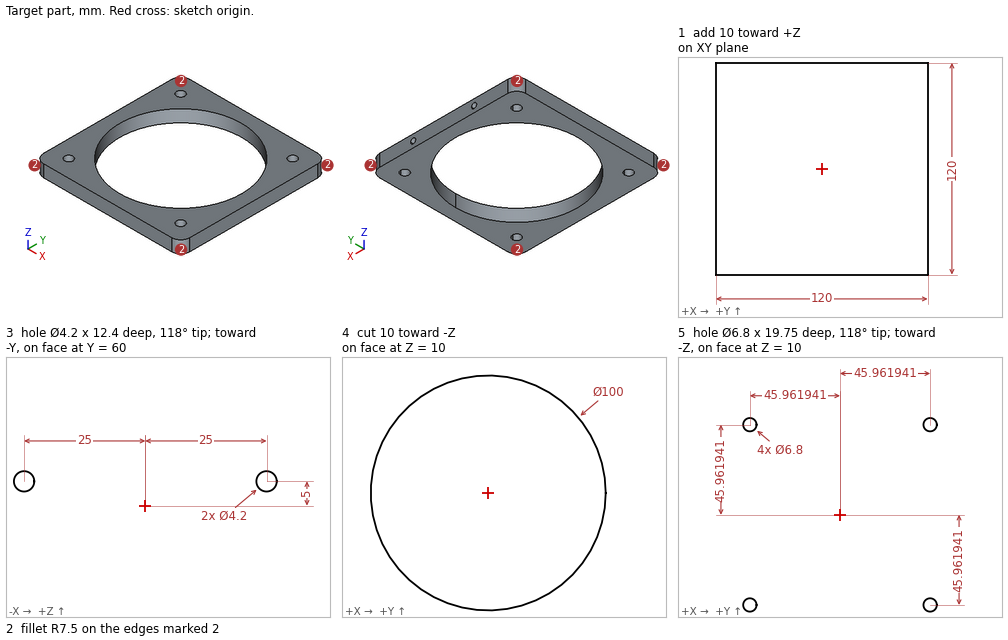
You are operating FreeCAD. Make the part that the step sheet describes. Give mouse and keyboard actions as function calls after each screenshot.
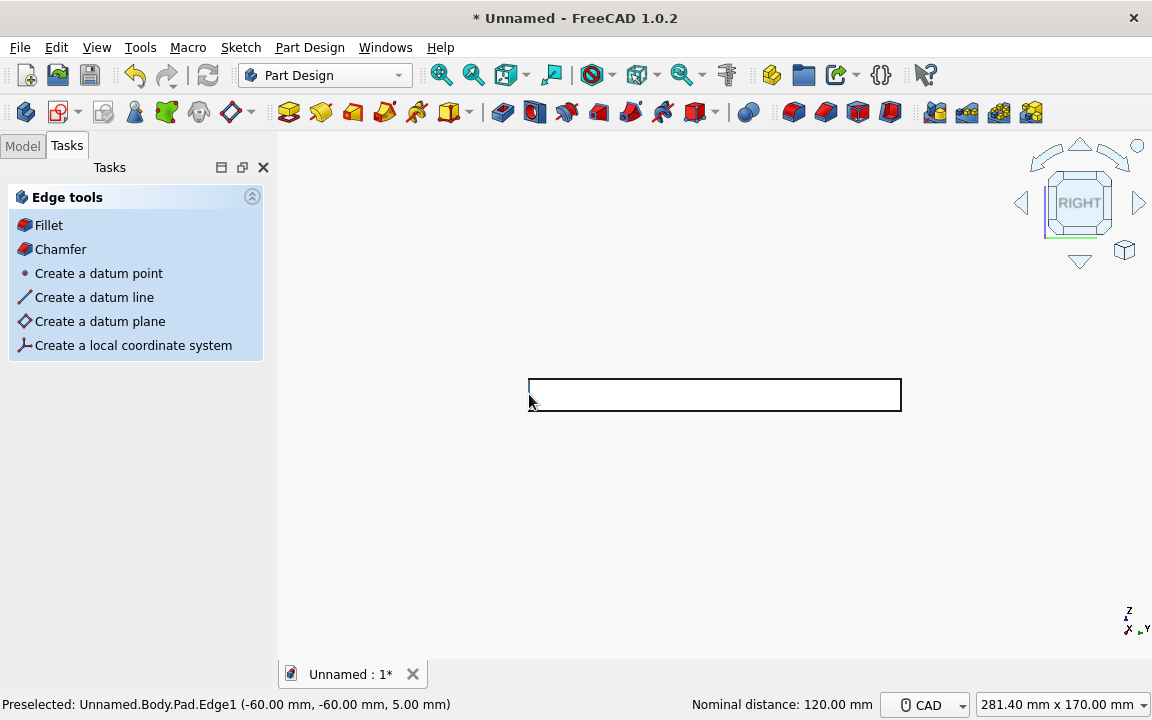
click(442, 76)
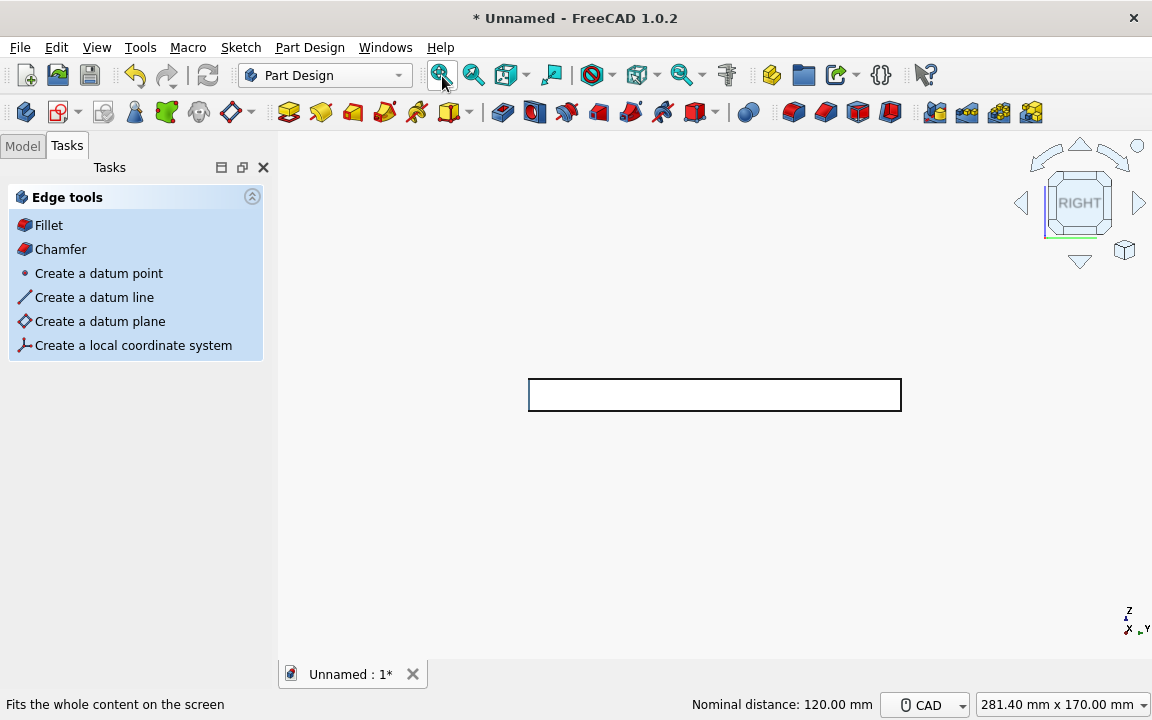
click(901, 394, ctrl)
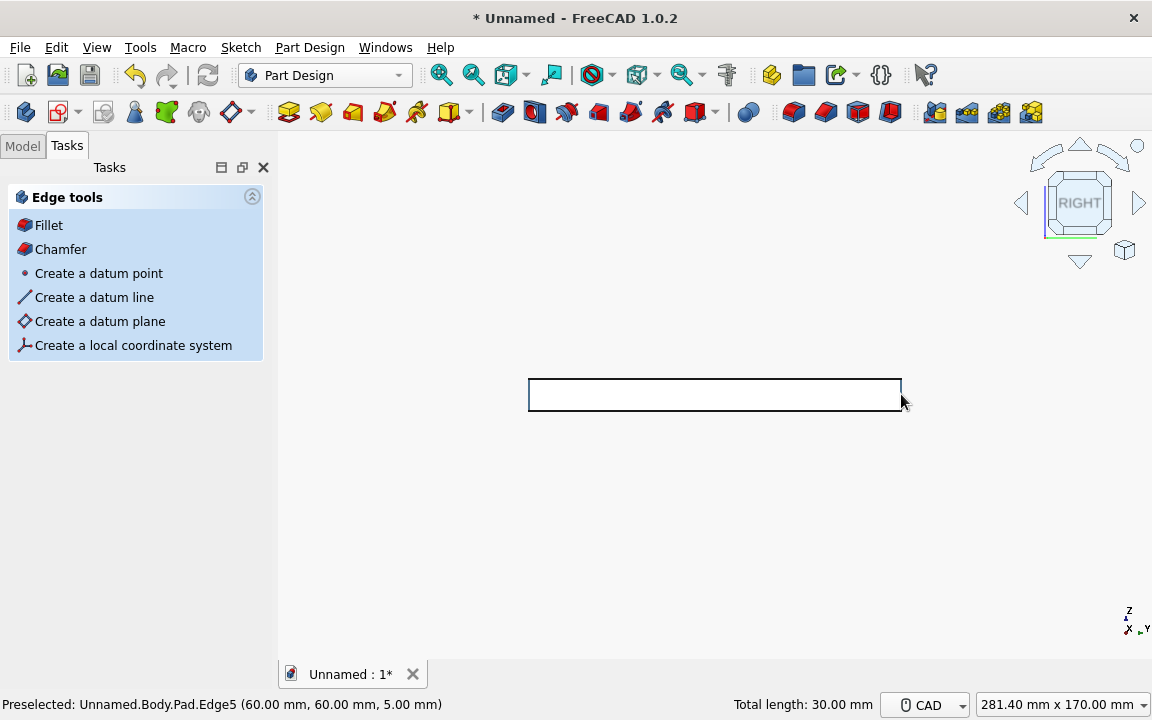
key(5)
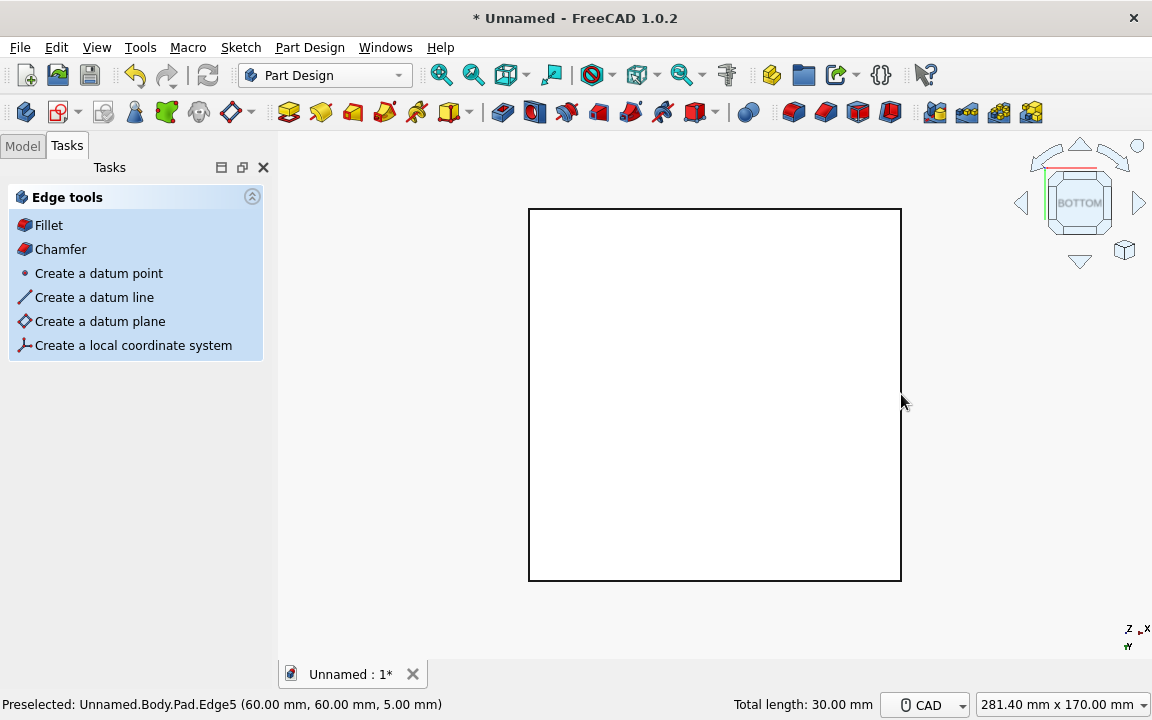
key(4)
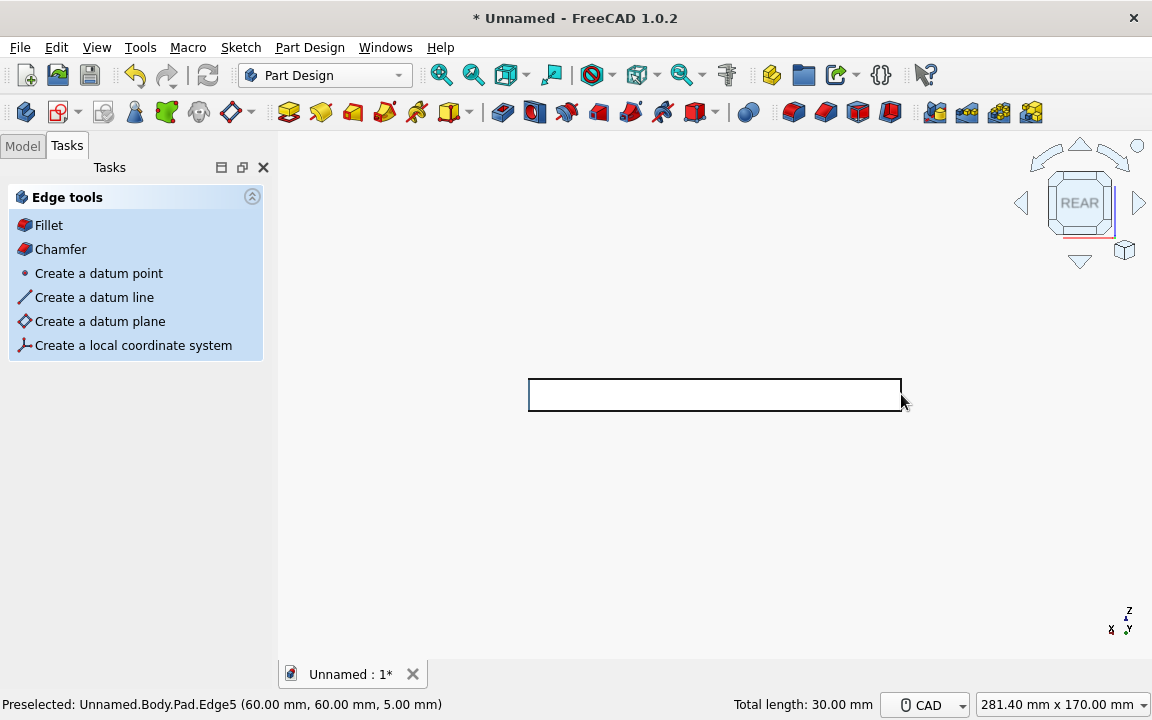
click(442, 76)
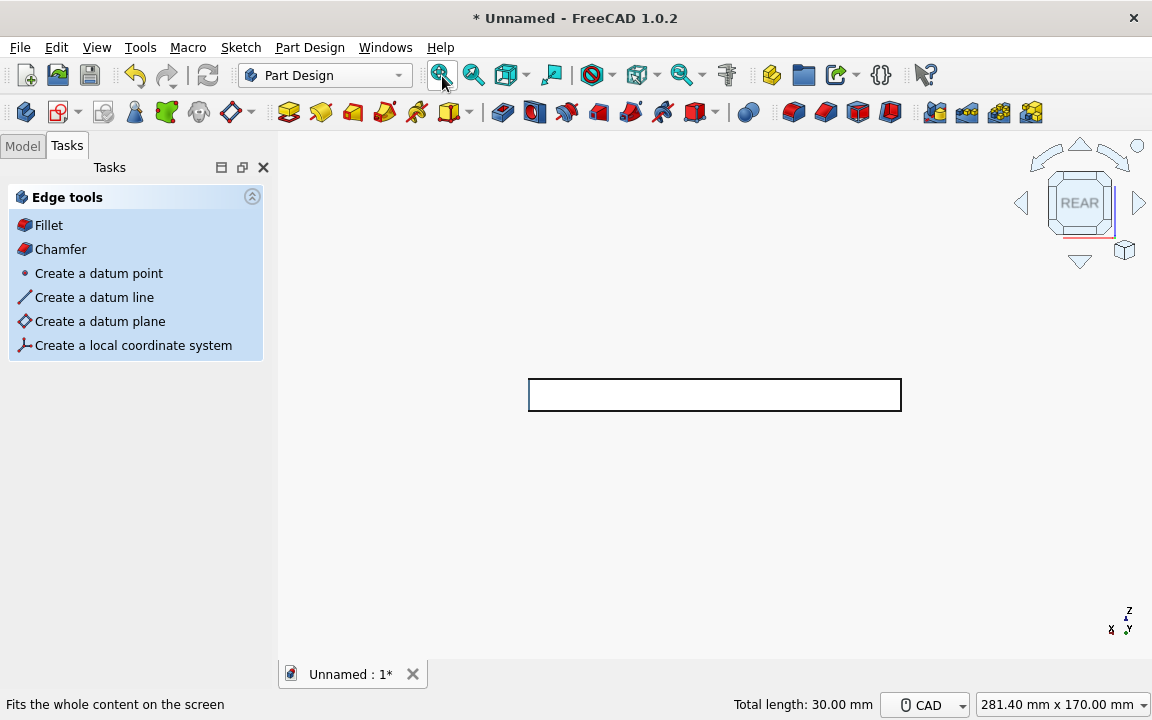
click(901, 394, ctrl)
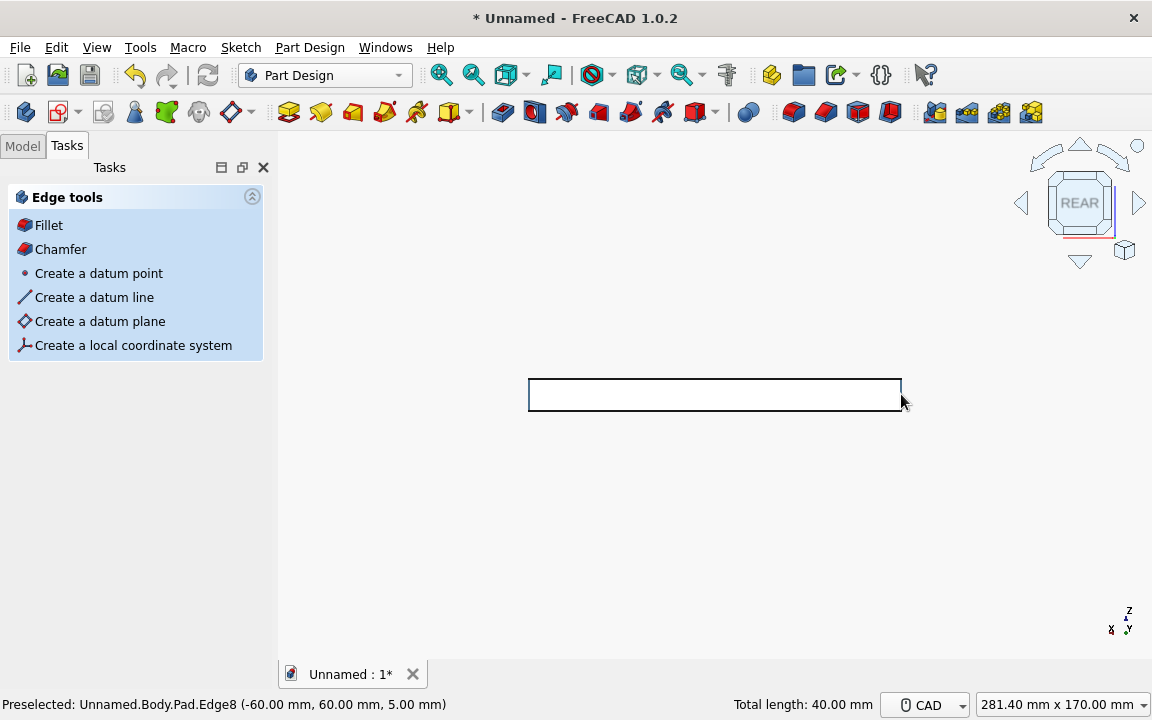
click(794, 112)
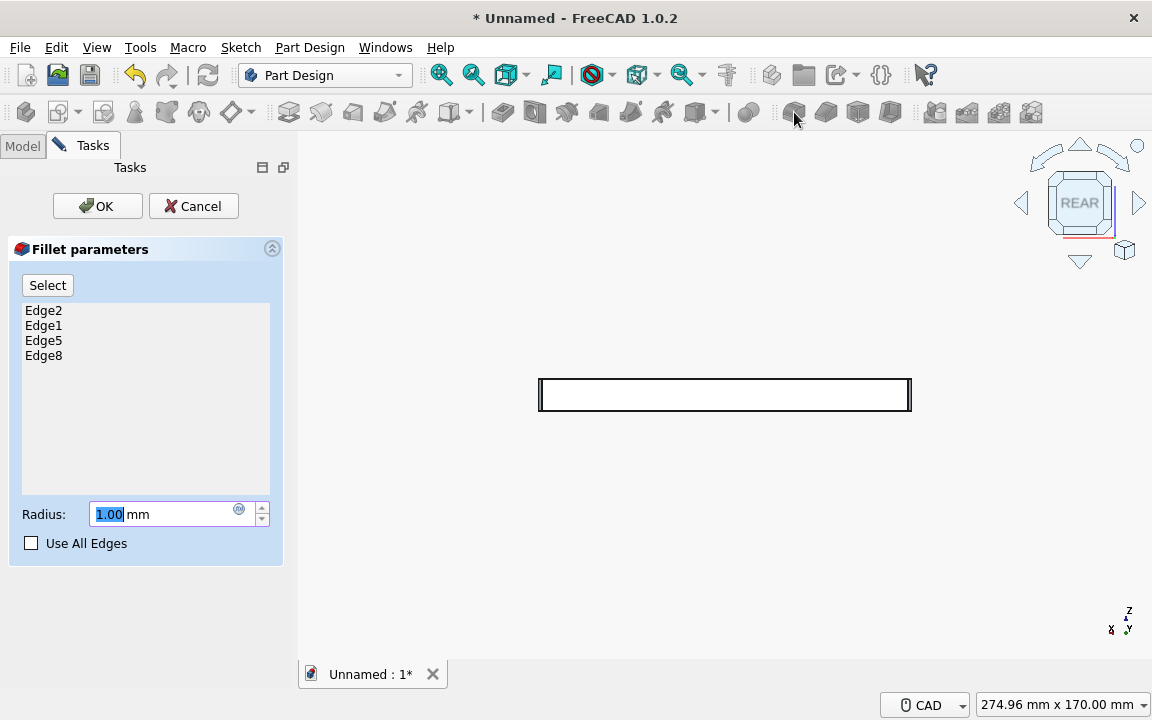
text(7.5)
key(Tab)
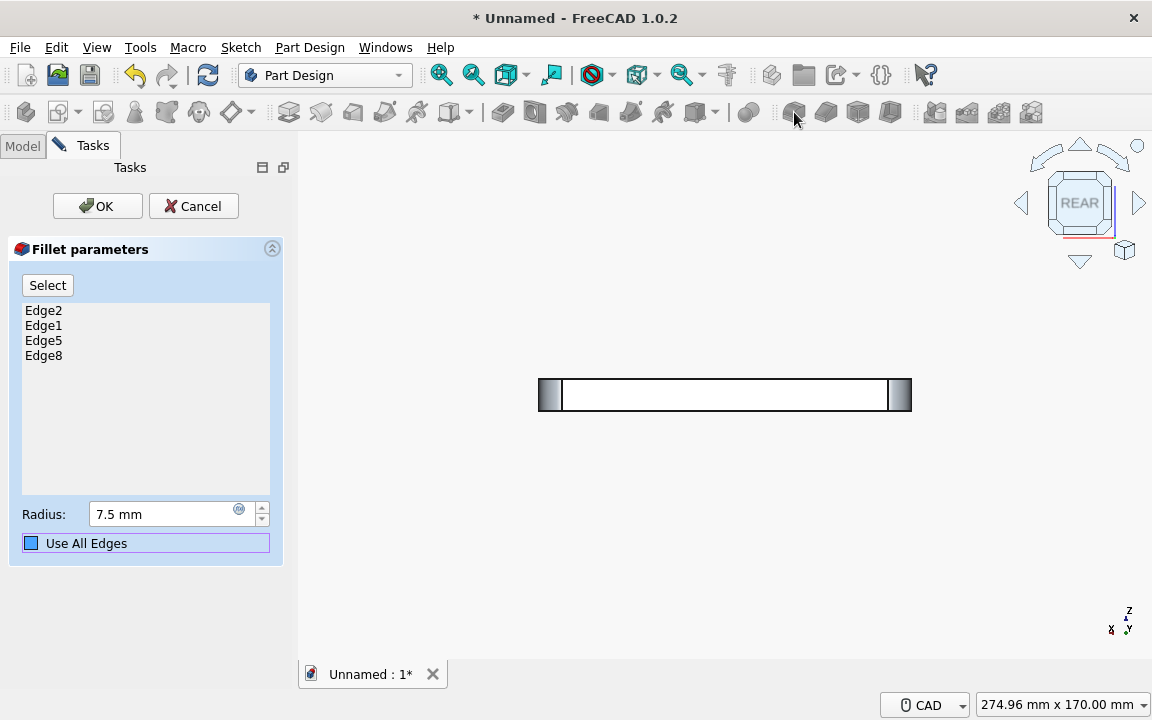
click(98, 206)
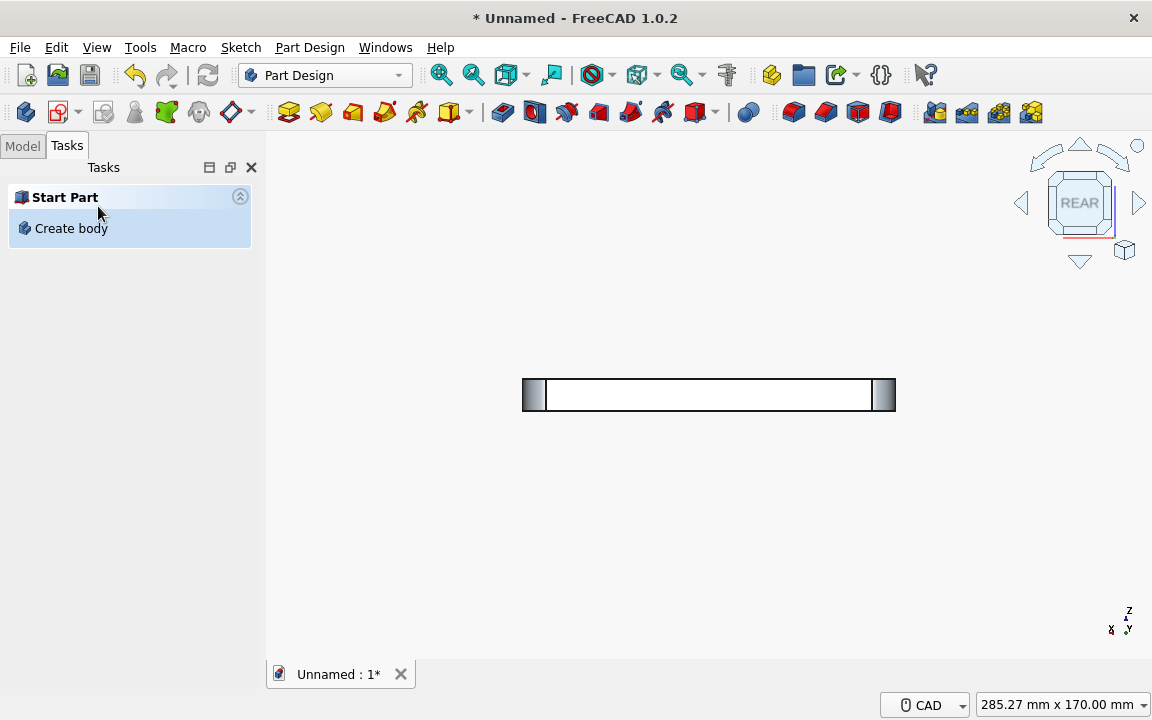
click(442, 76)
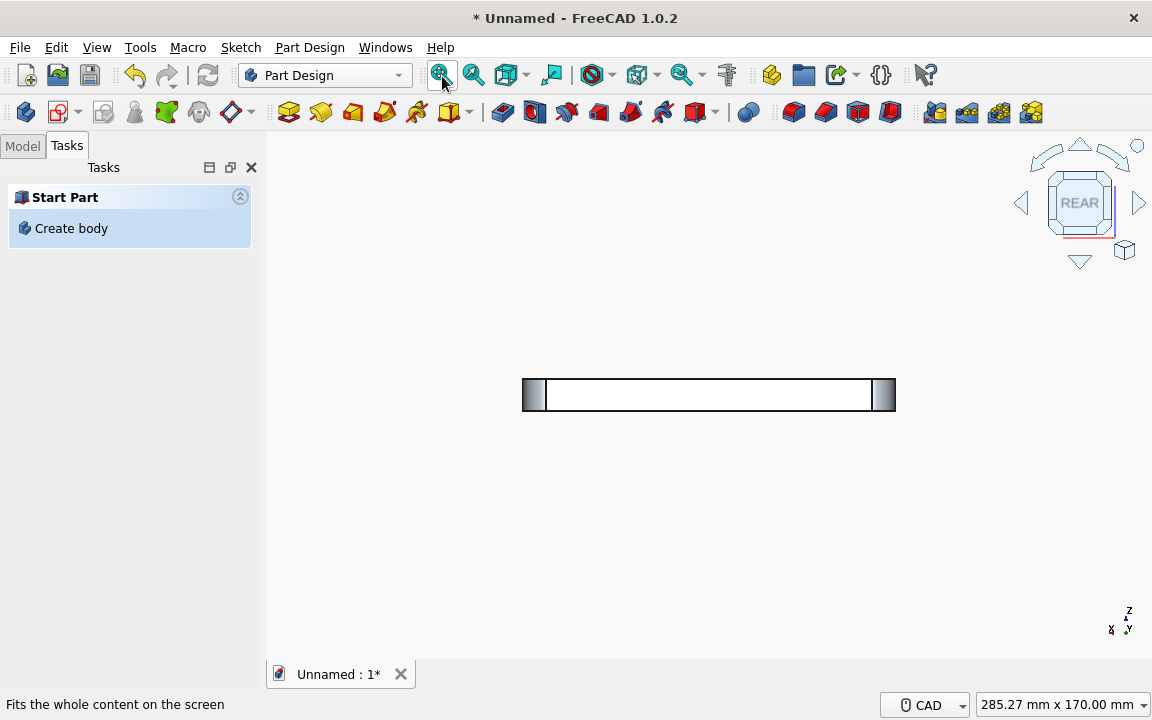
click(569, 394)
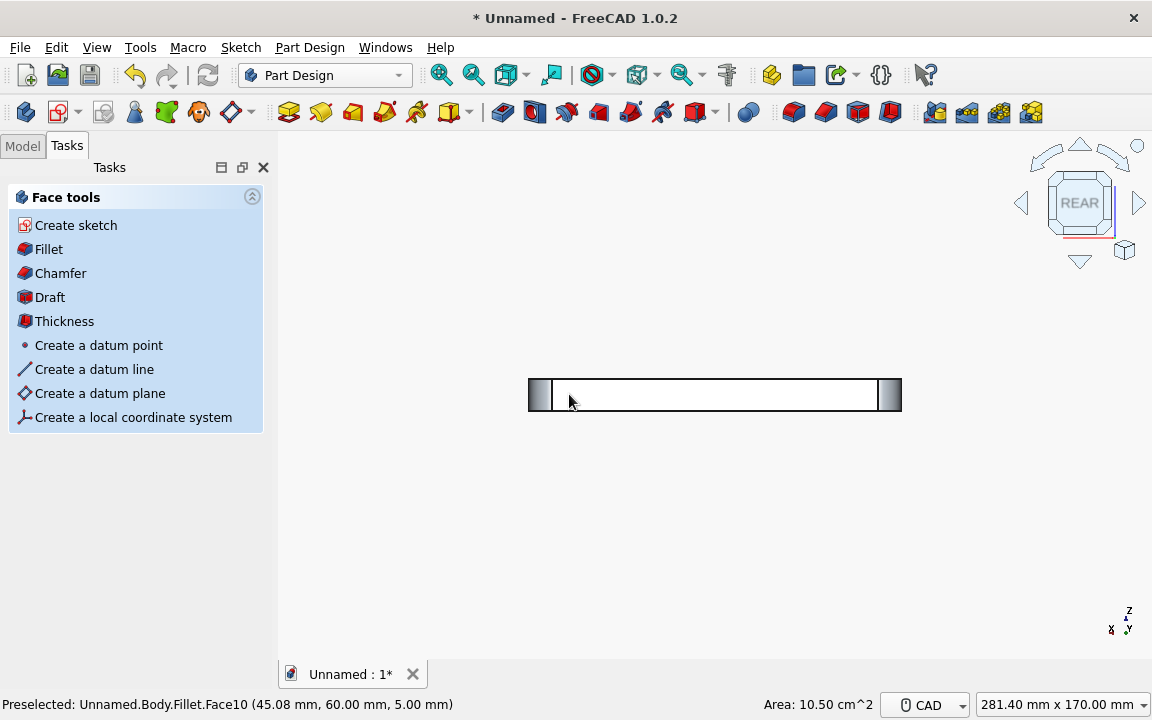
click(58, 112)